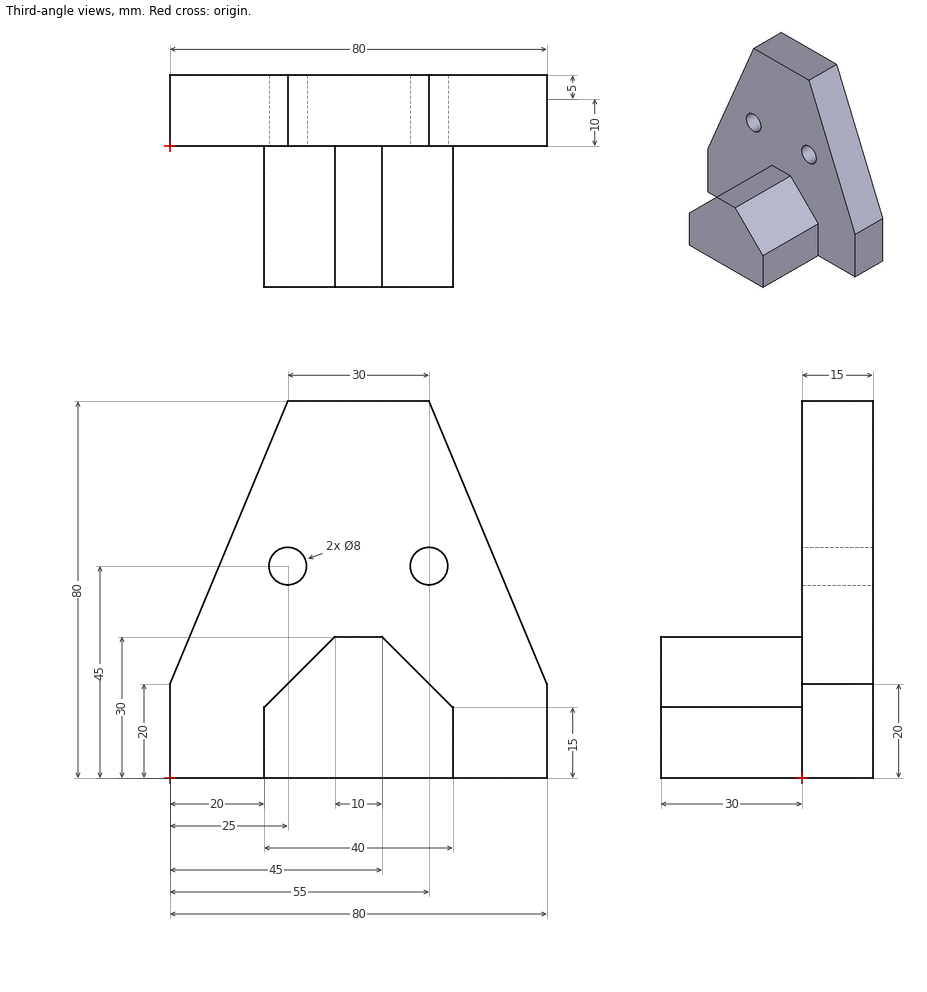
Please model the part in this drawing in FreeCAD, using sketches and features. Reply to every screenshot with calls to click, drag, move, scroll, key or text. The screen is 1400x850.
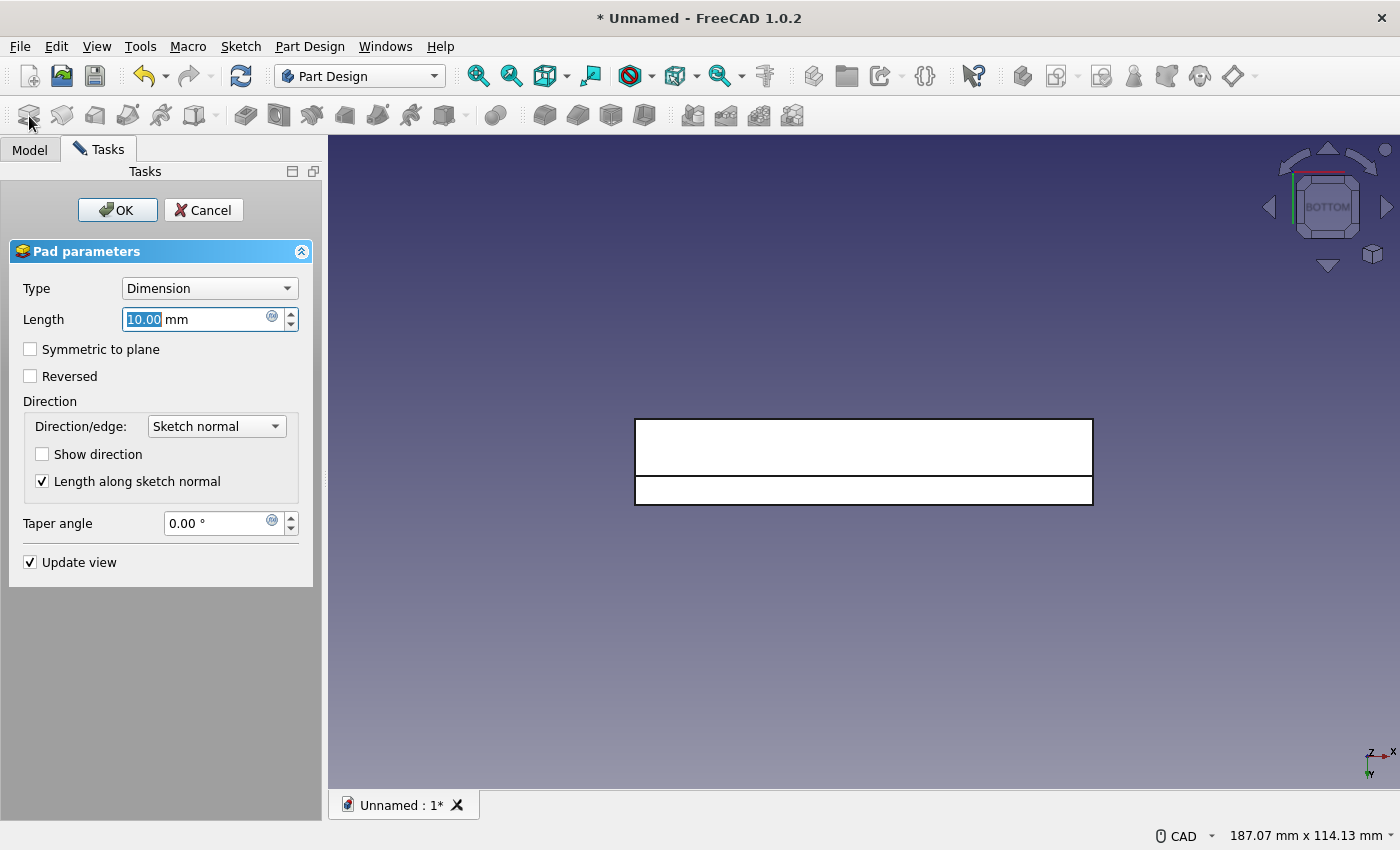
text(20)
key(Tab)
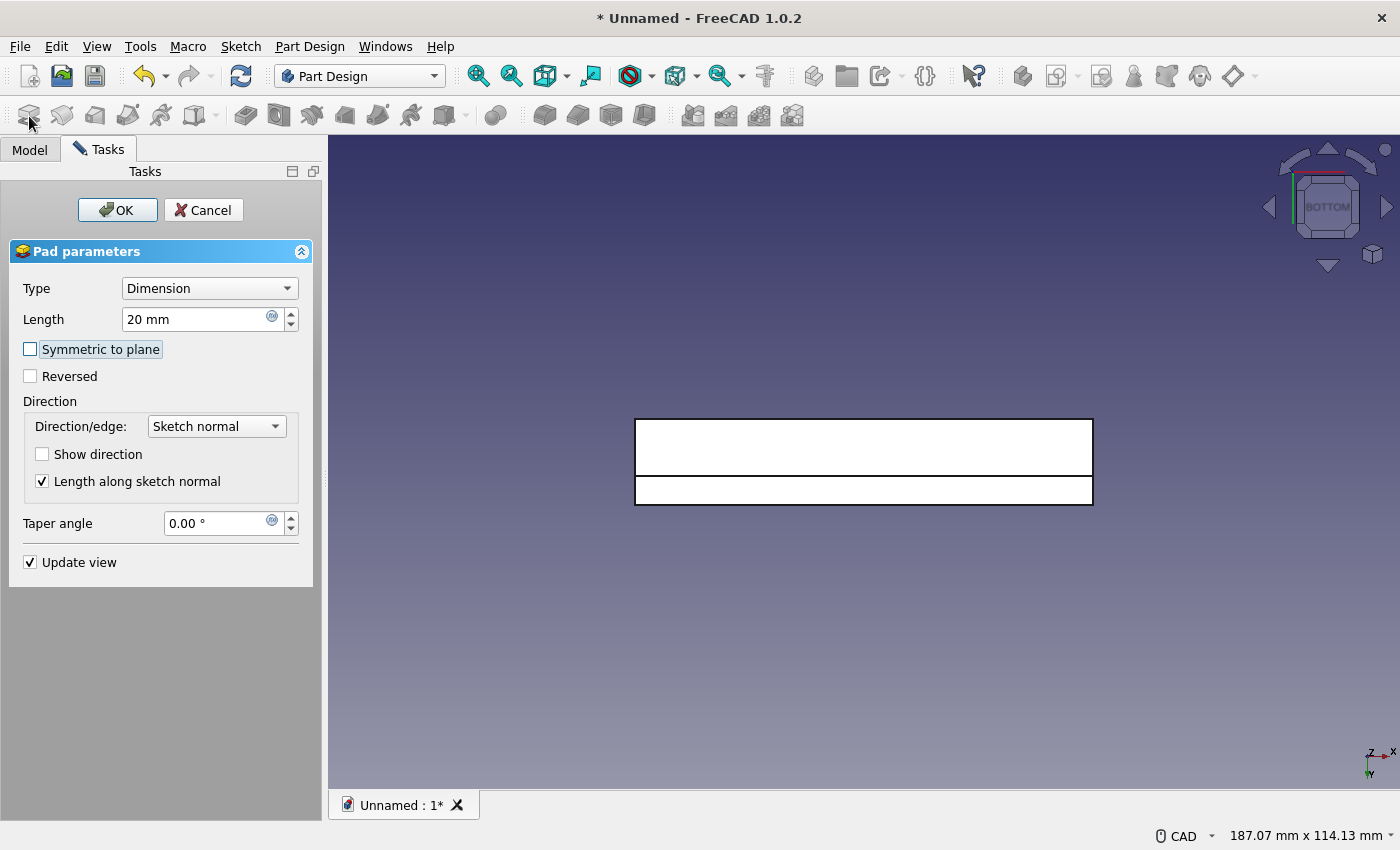
click(31, 376)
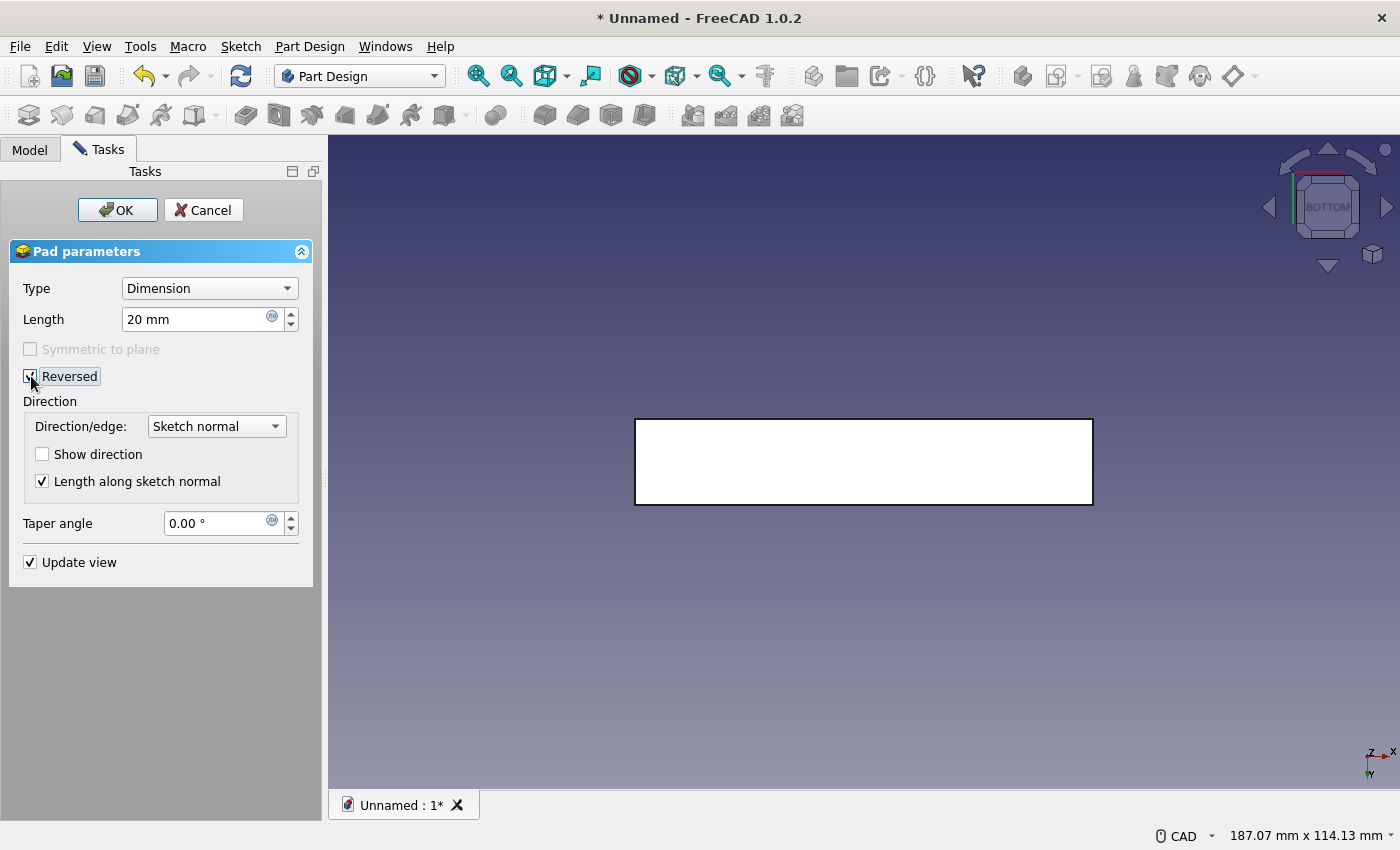
click(118, 210)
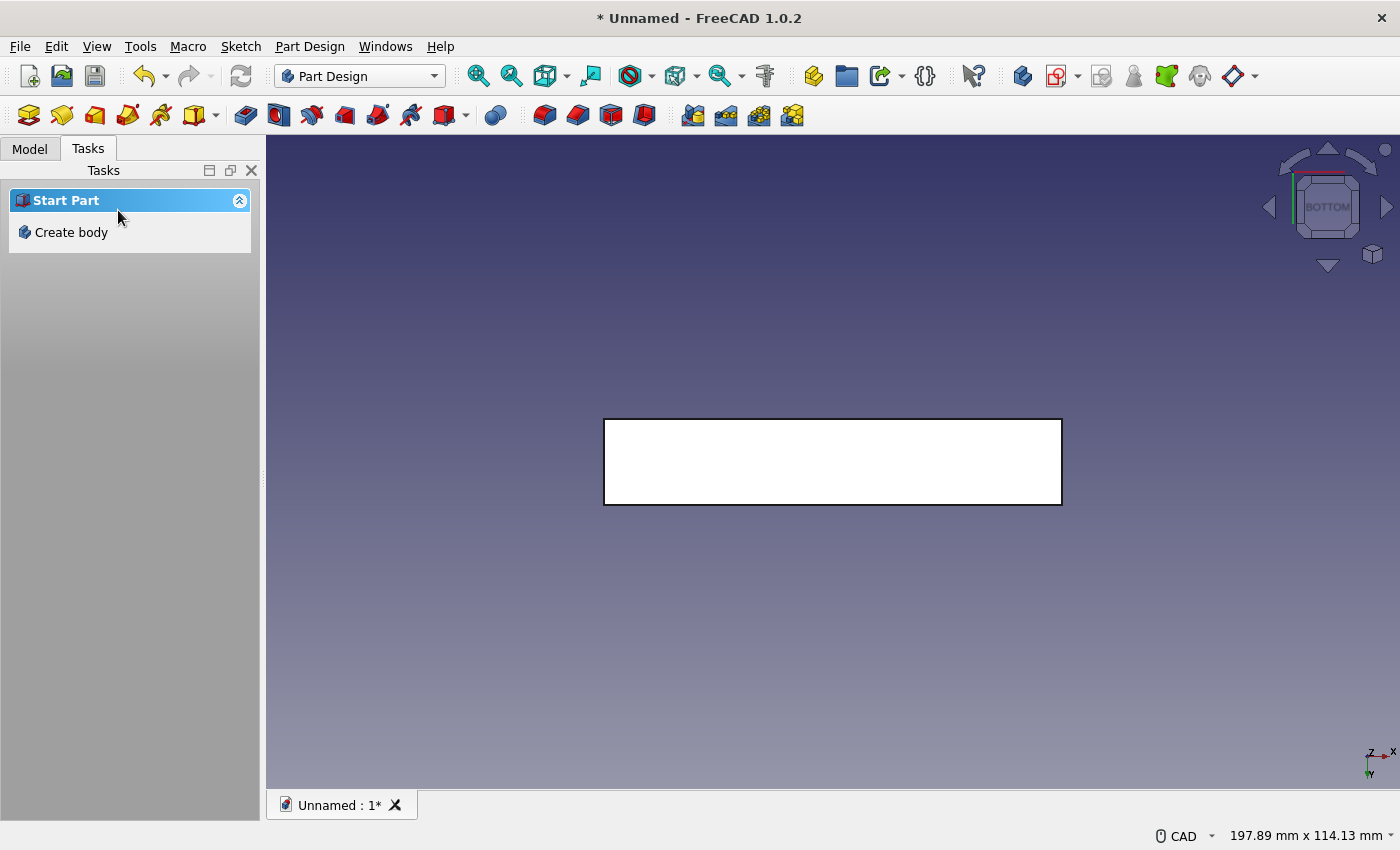
key(v)
key(f)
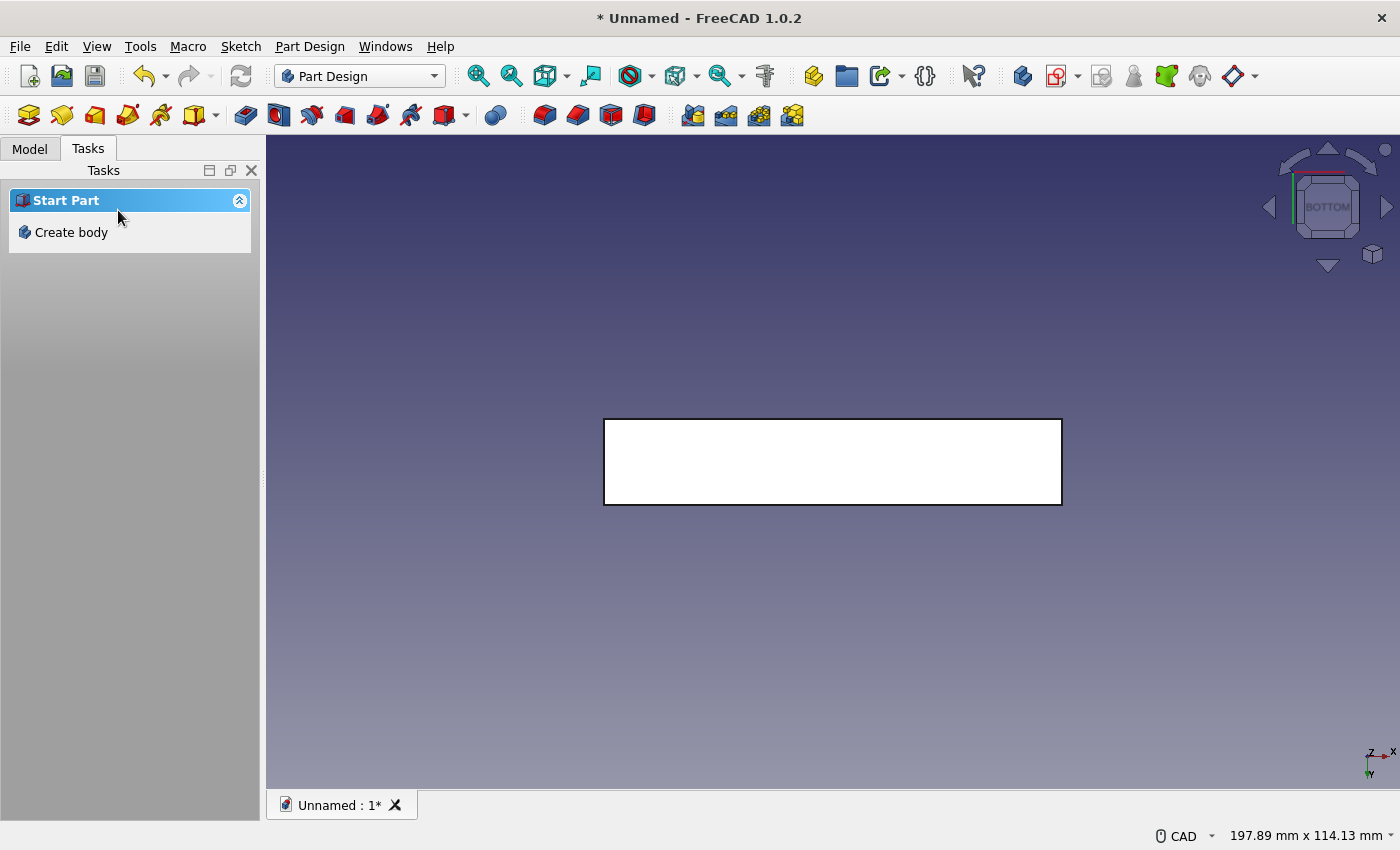
click(1056, 76)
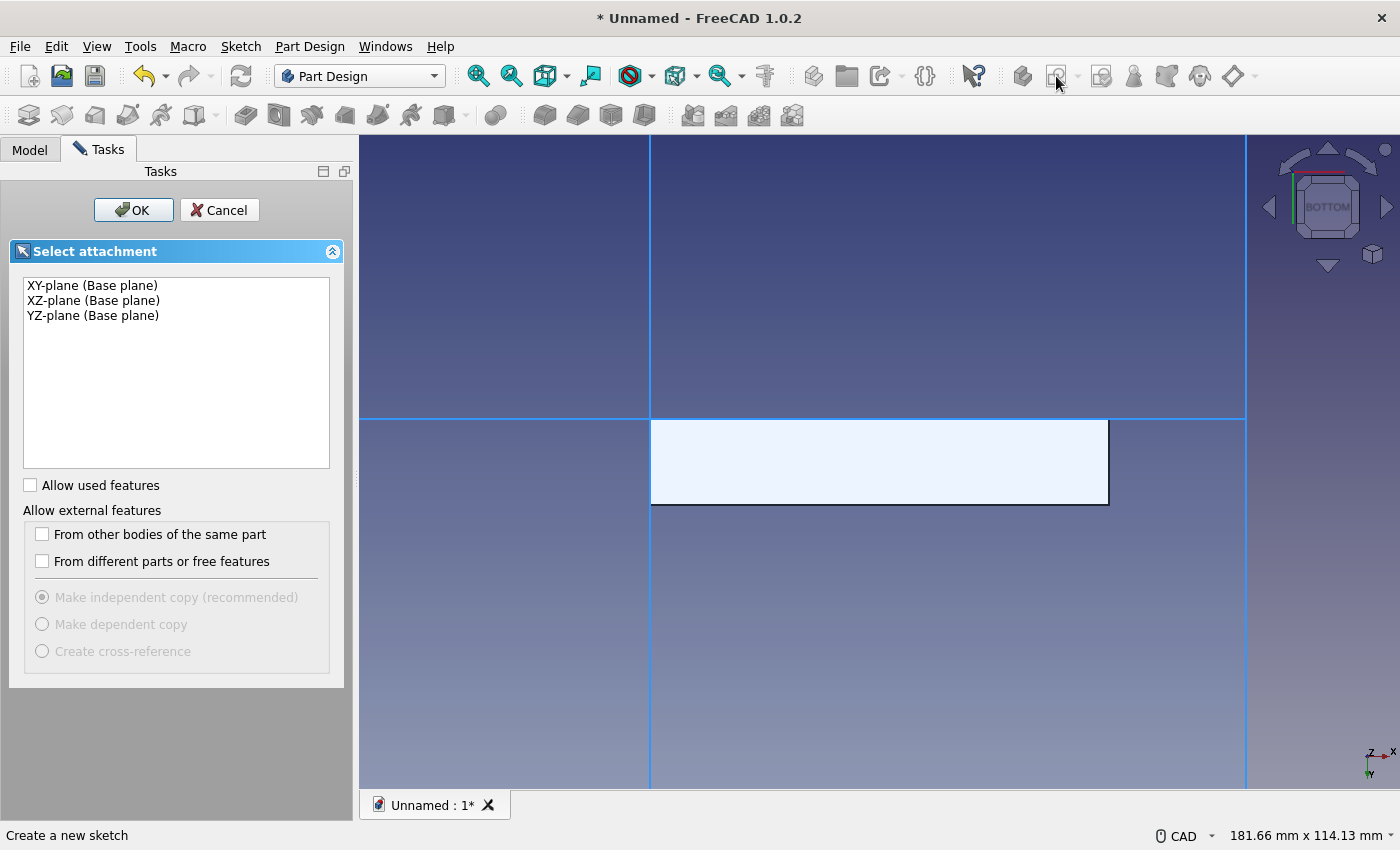
click(84, 300)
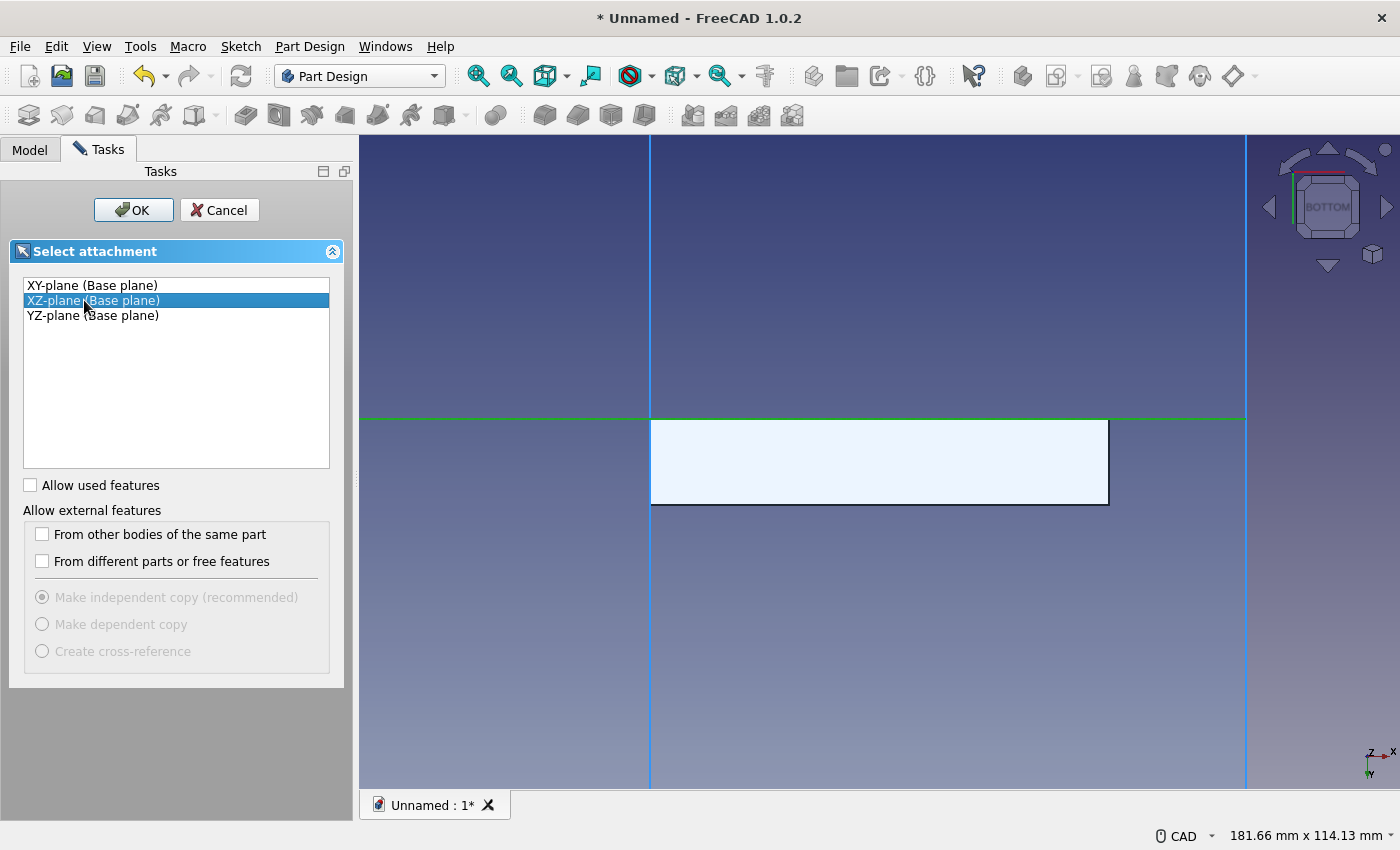
click(134, 210)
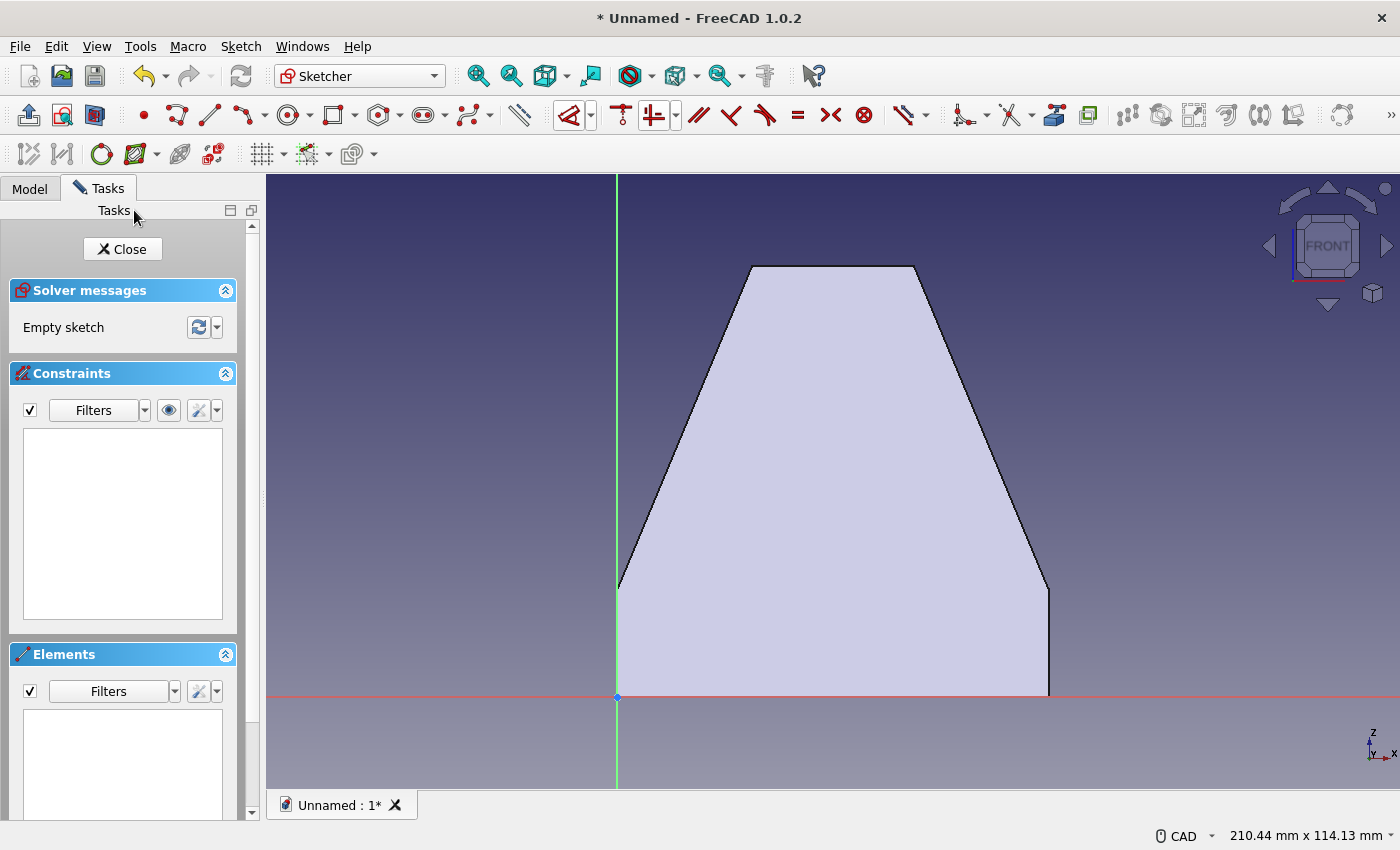
scroll(791, 726, up, 4)